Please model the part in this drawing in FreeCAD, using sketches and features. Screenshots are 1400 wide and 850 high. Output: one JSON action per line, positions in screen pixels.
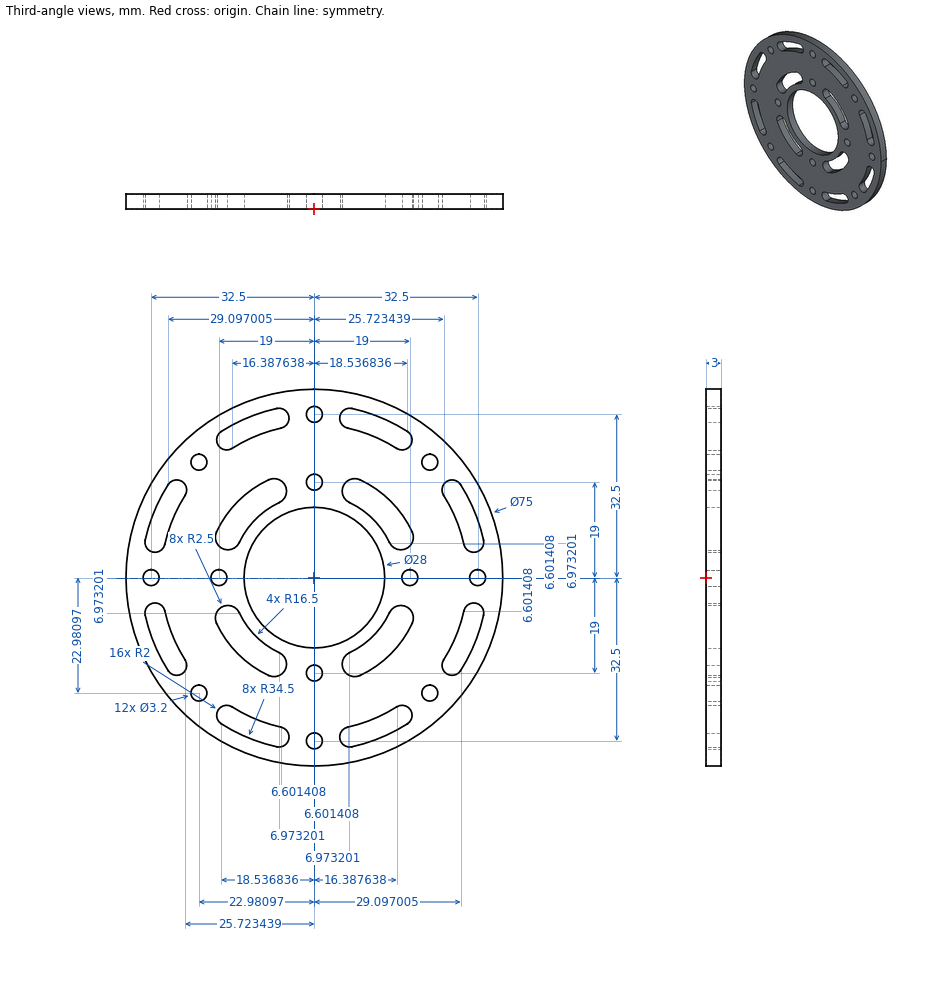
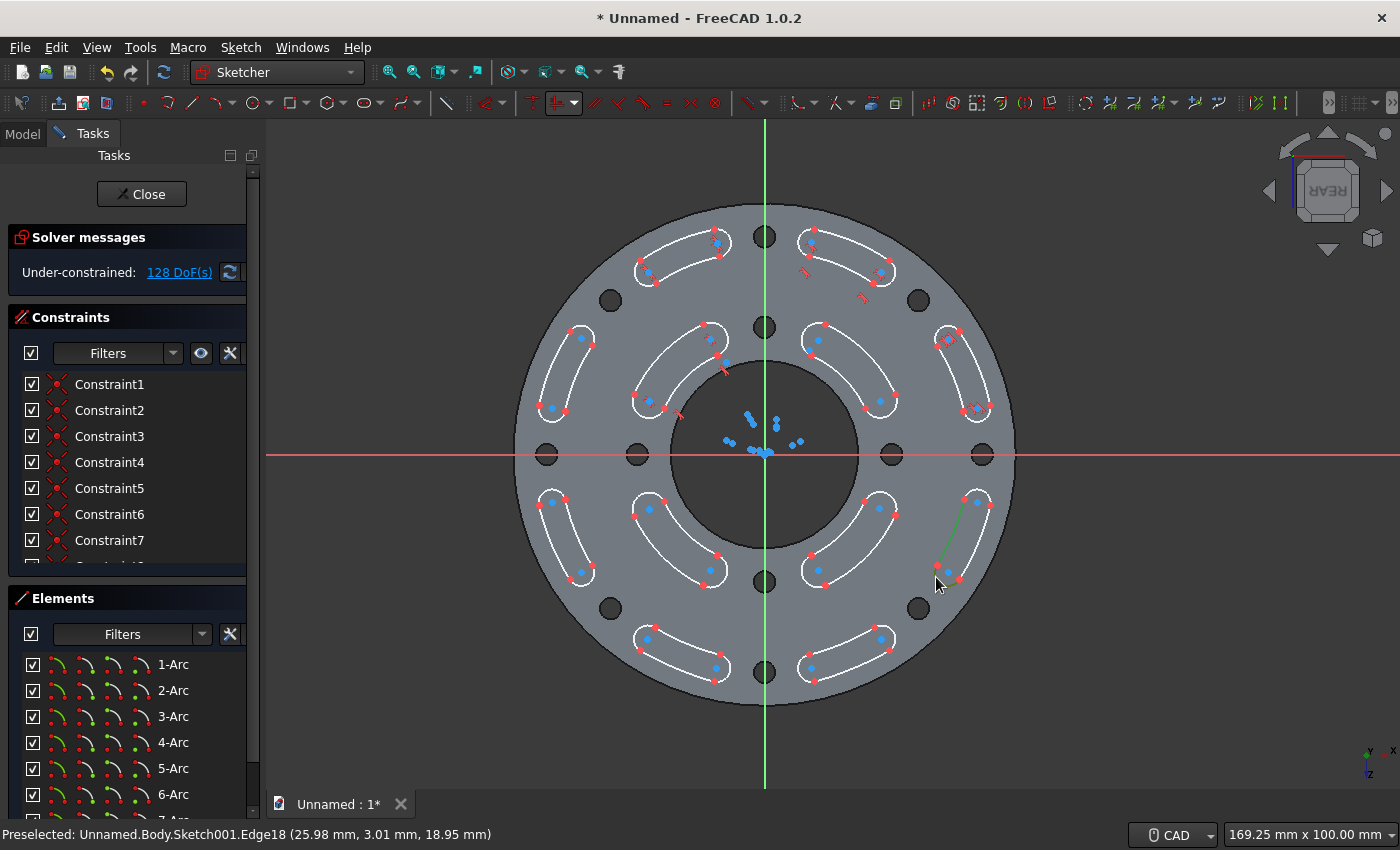
{"action": "left_click", "coordinate": [644, 104]}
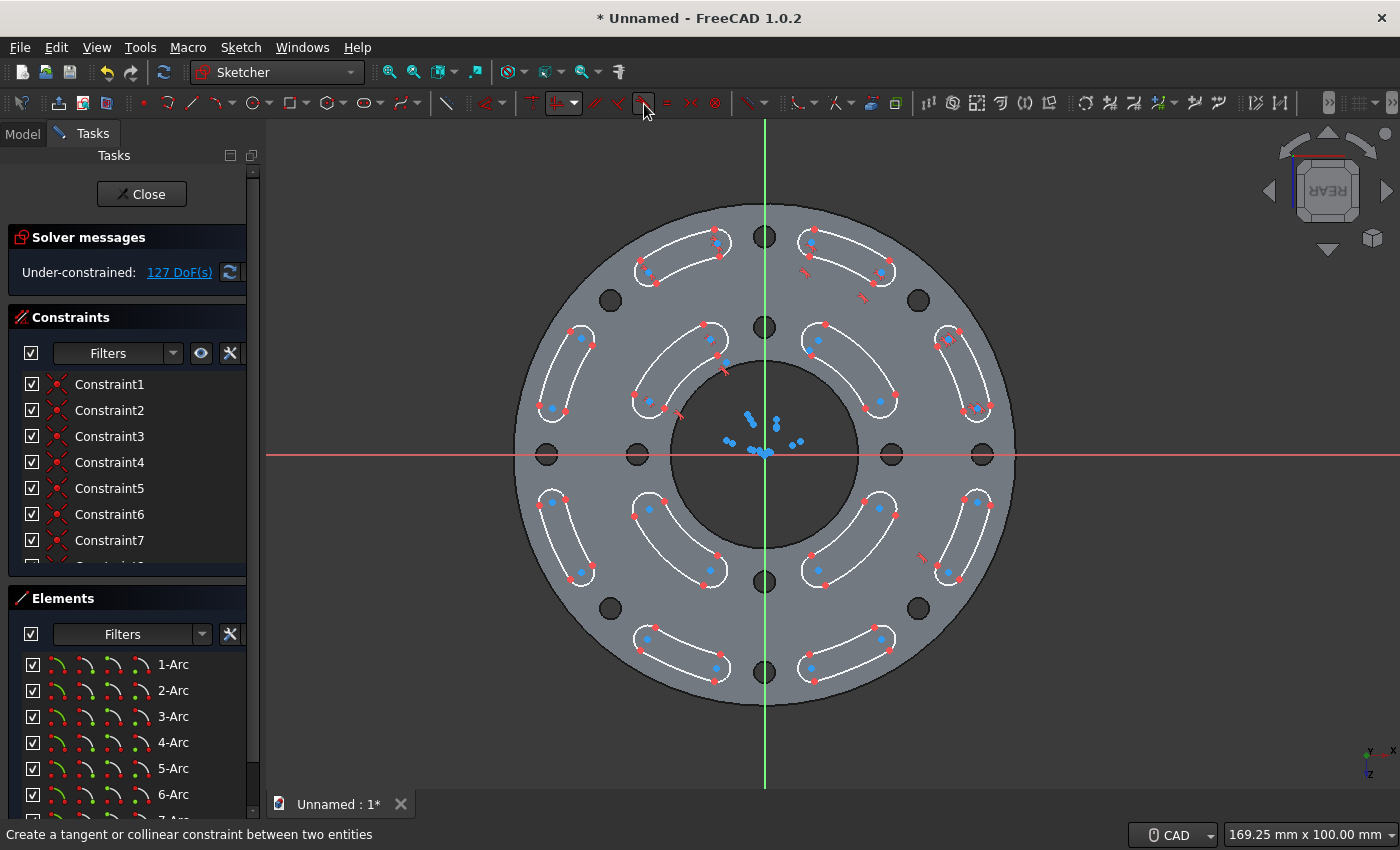
{"action": "left_click", "coordinate": [947, 547]}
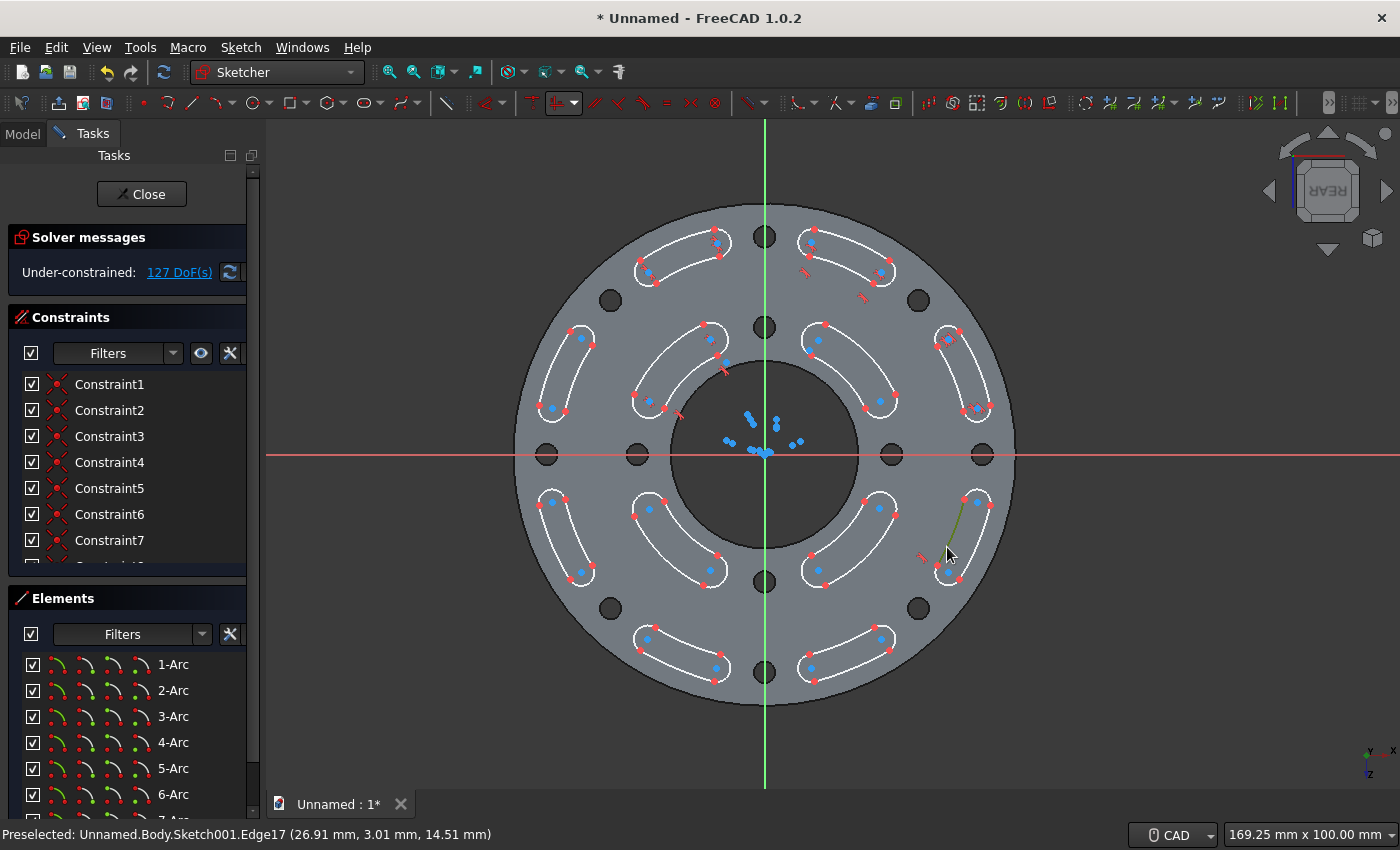
{"action": "left_click", "coordinate": [987, 494]}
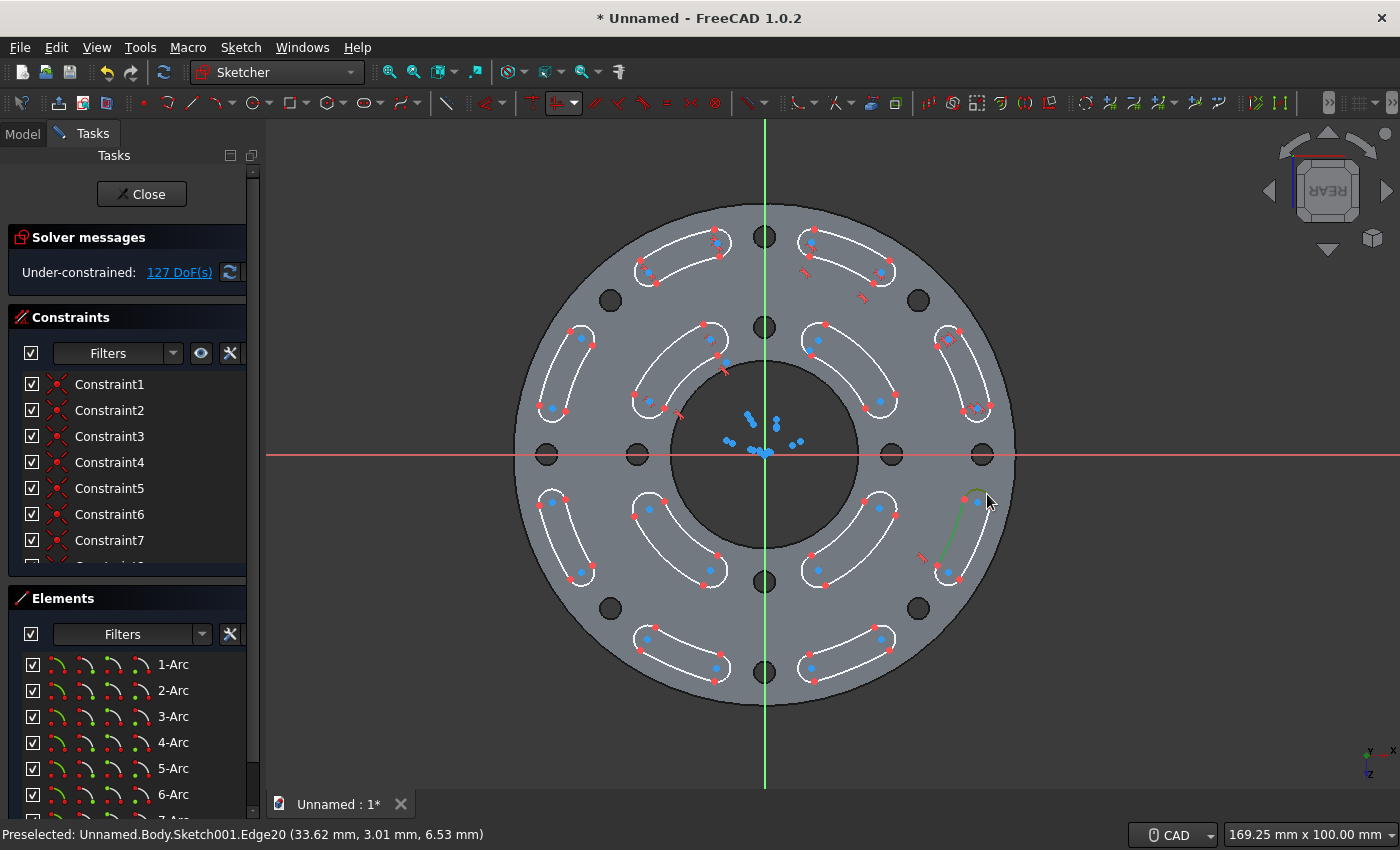
{"action": "left_click", "coordinate": [644, 104]}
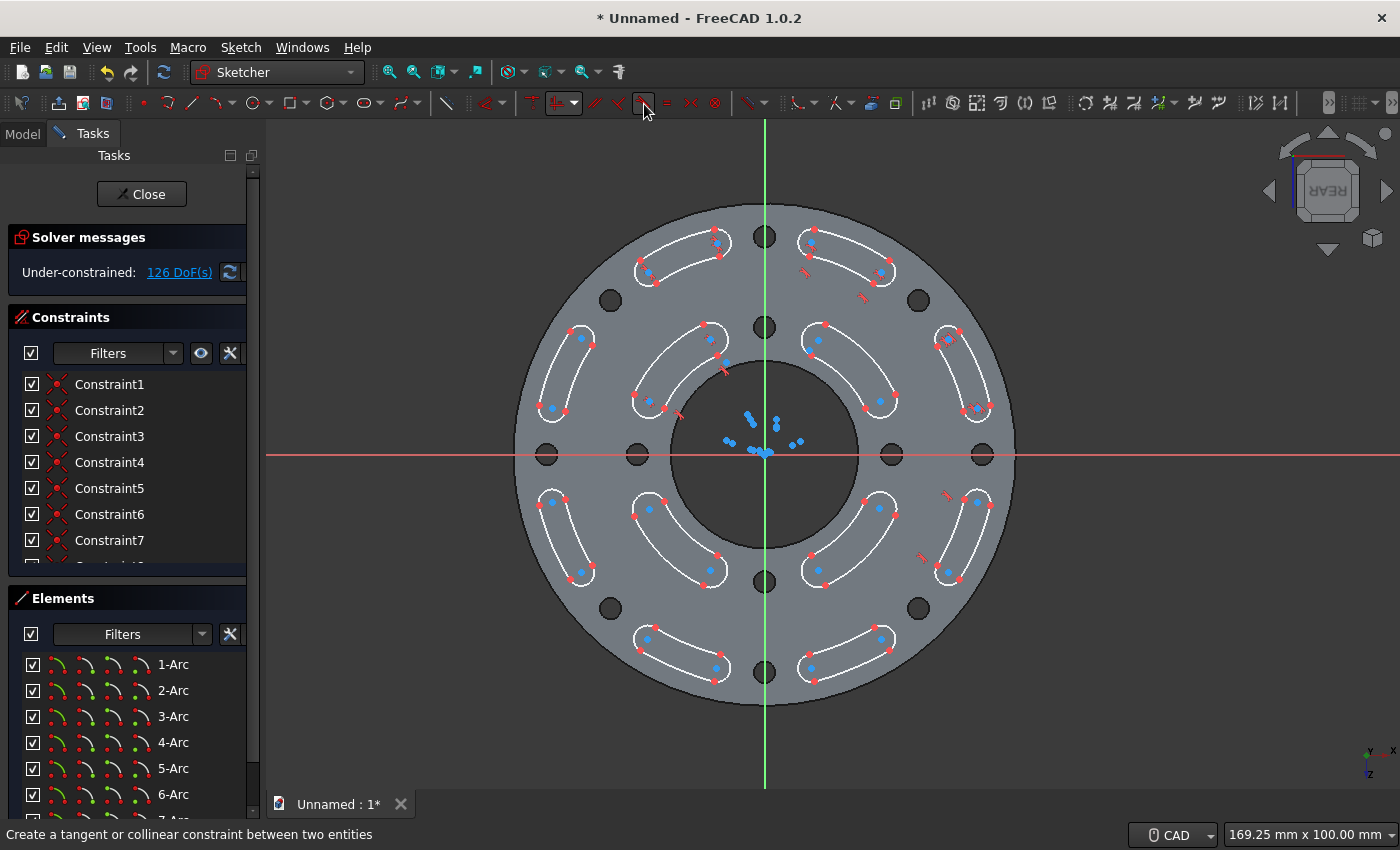
{"action": "left_click", "coordinate": [936, 577]}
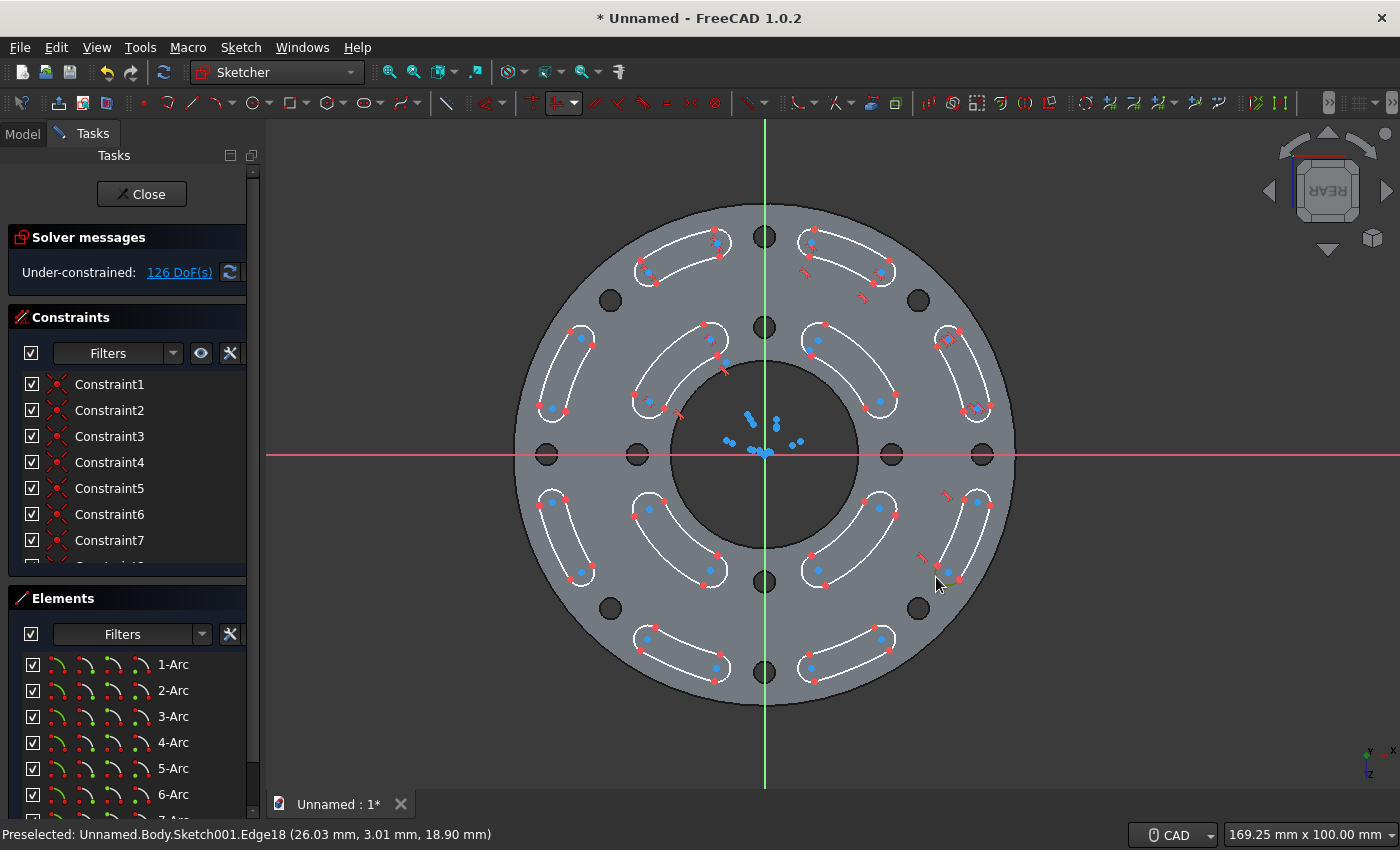
{"action": "left_click", "coordinate": [971, 559]}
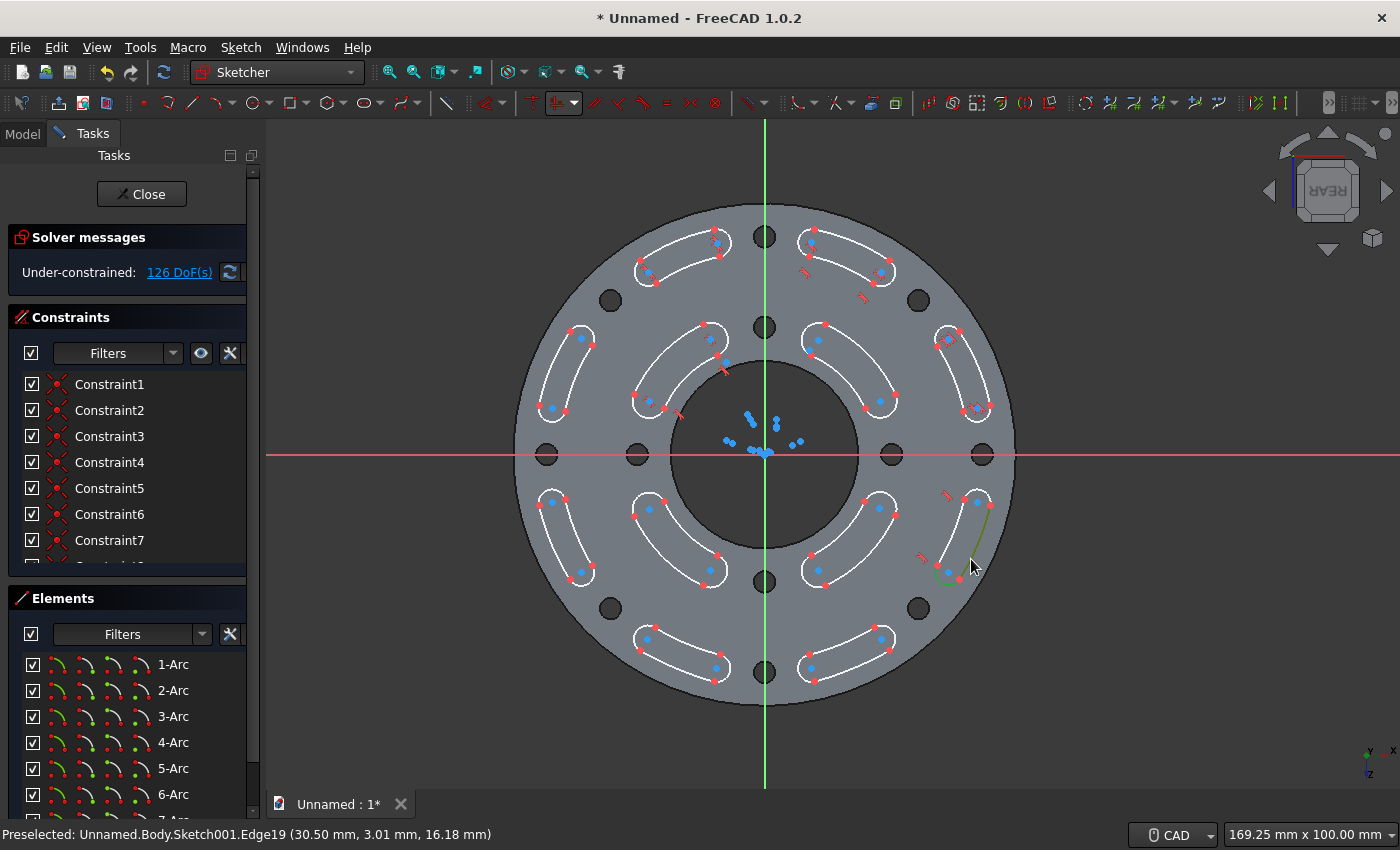
{"action": "left_click", "coordinate": [644, 104]}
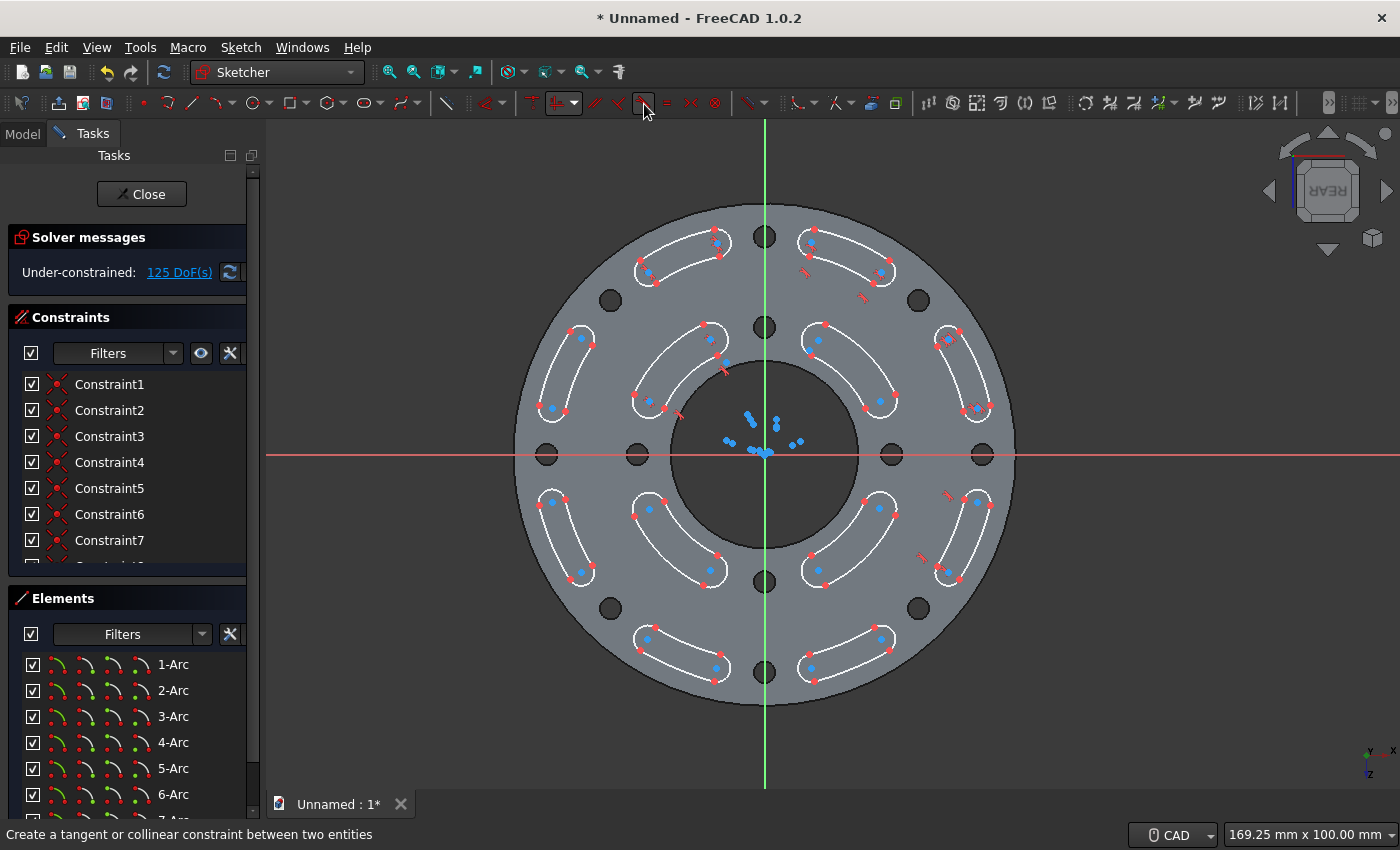
{"action": "left_click", "coordinate": [971, 559]}